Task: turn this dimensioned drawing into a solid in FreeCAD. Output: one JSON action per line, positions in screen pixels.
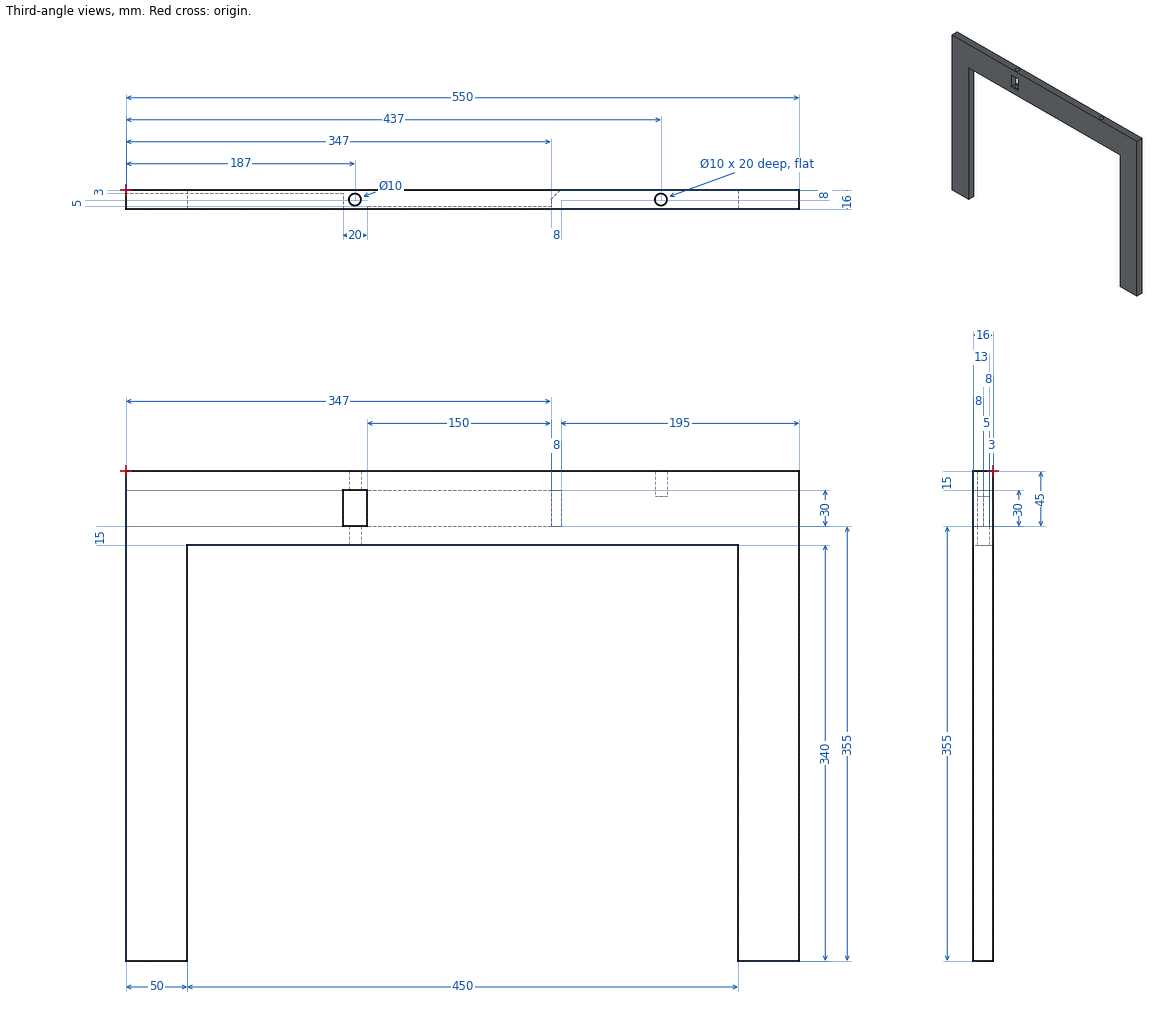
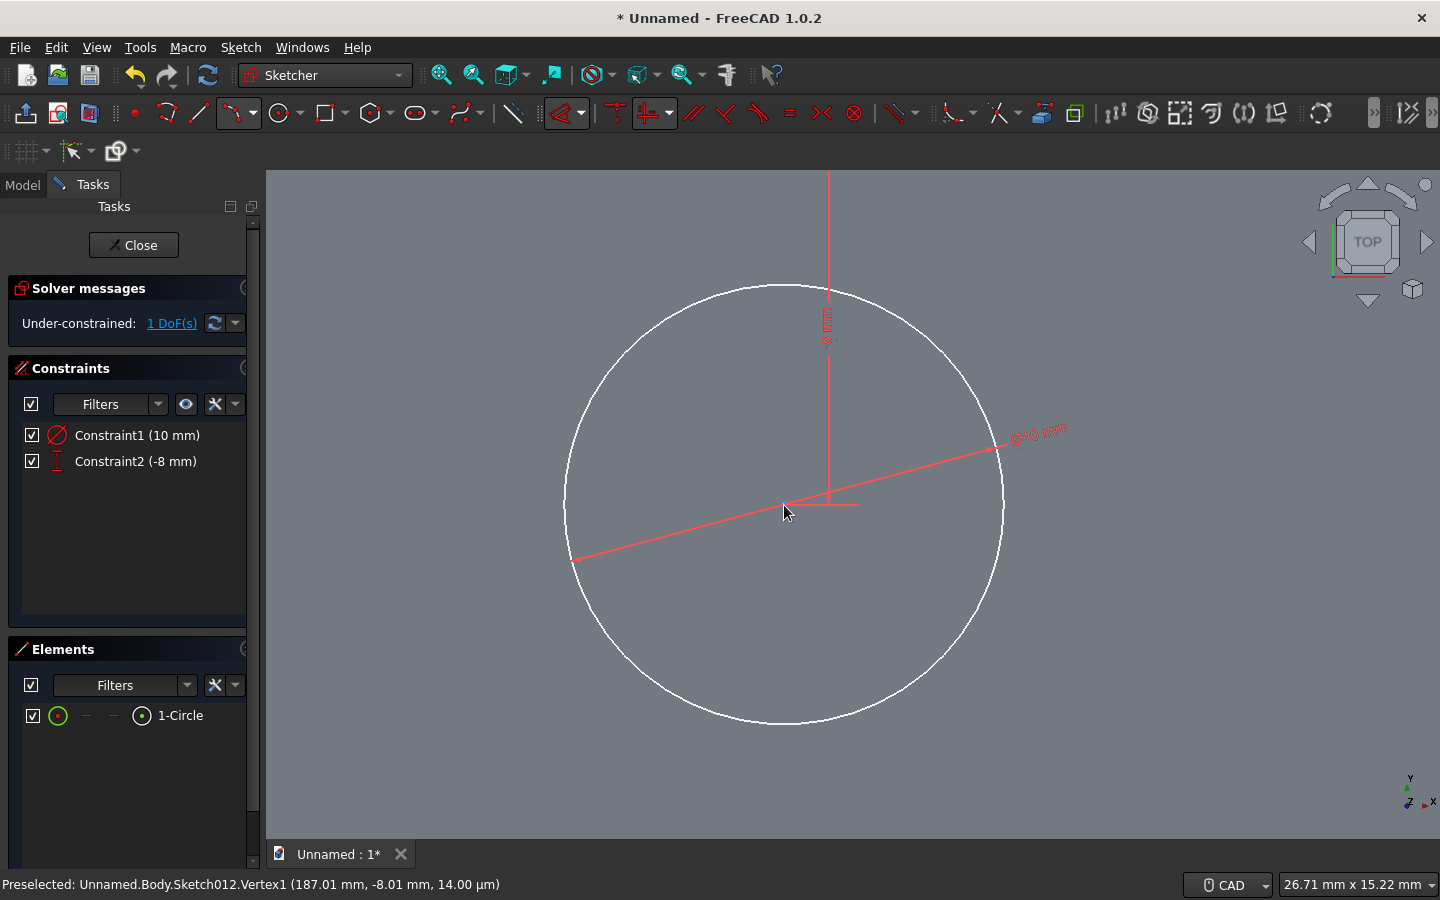
{"action": "left_click", "coordinate": [784, 504]}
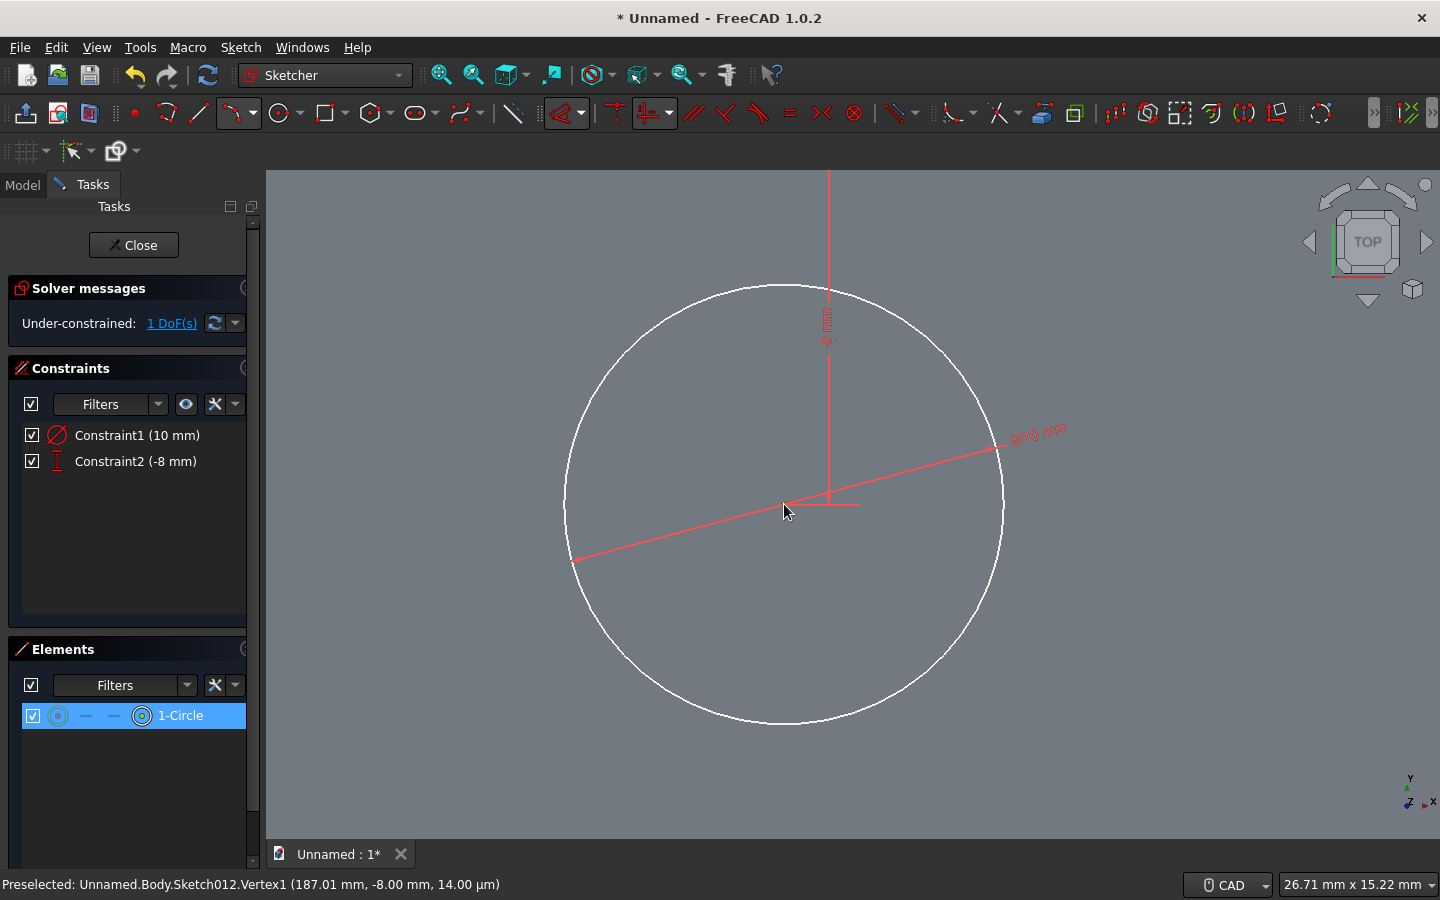
{"action": "key", "text": "l"}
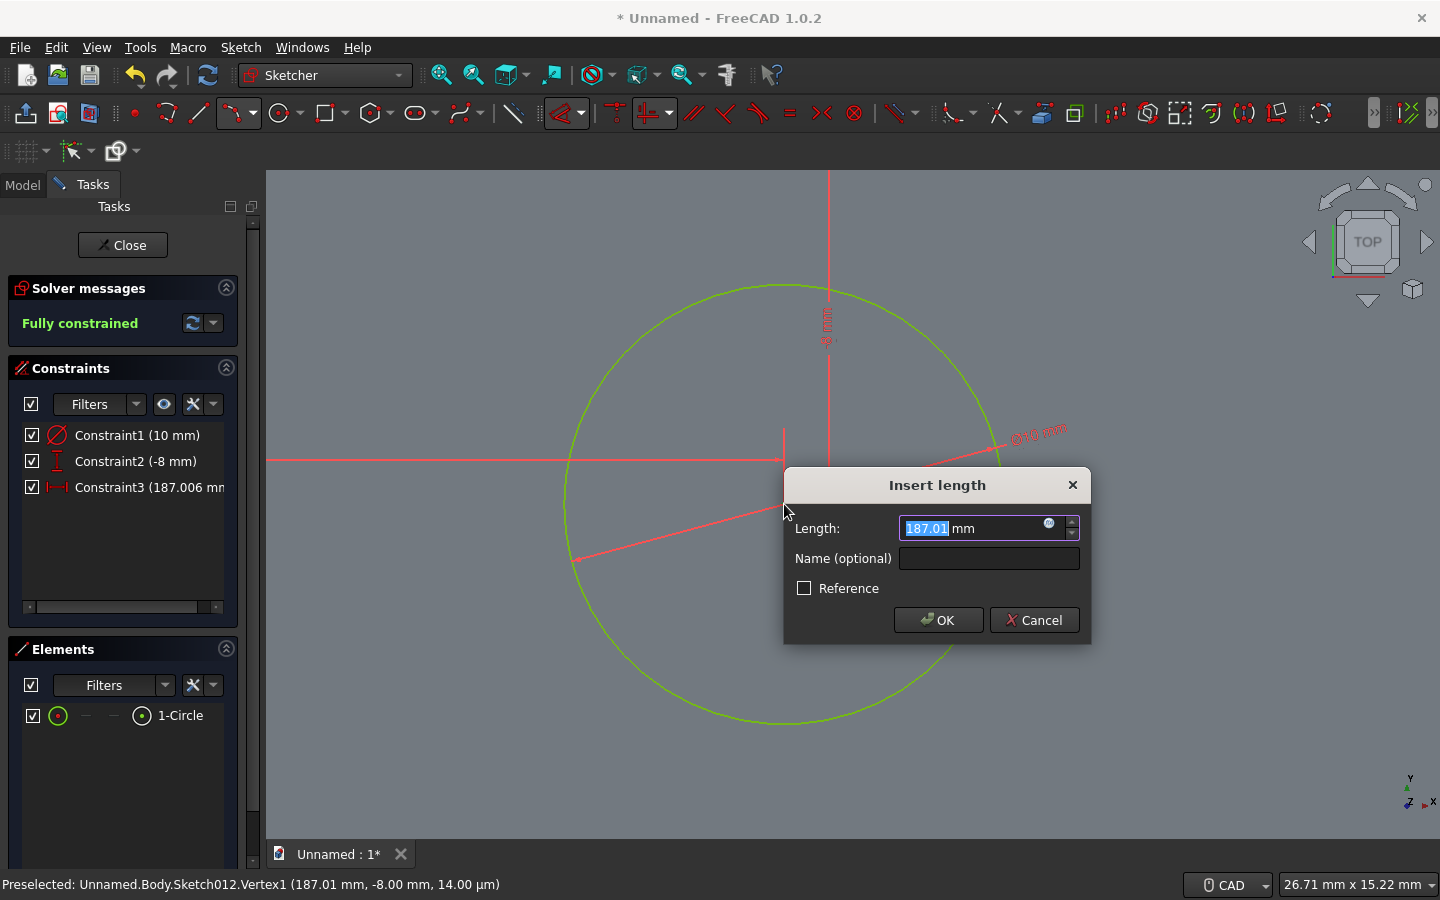
{"action": "type", "text": "187"}
{"action": "key", "text": "Return"}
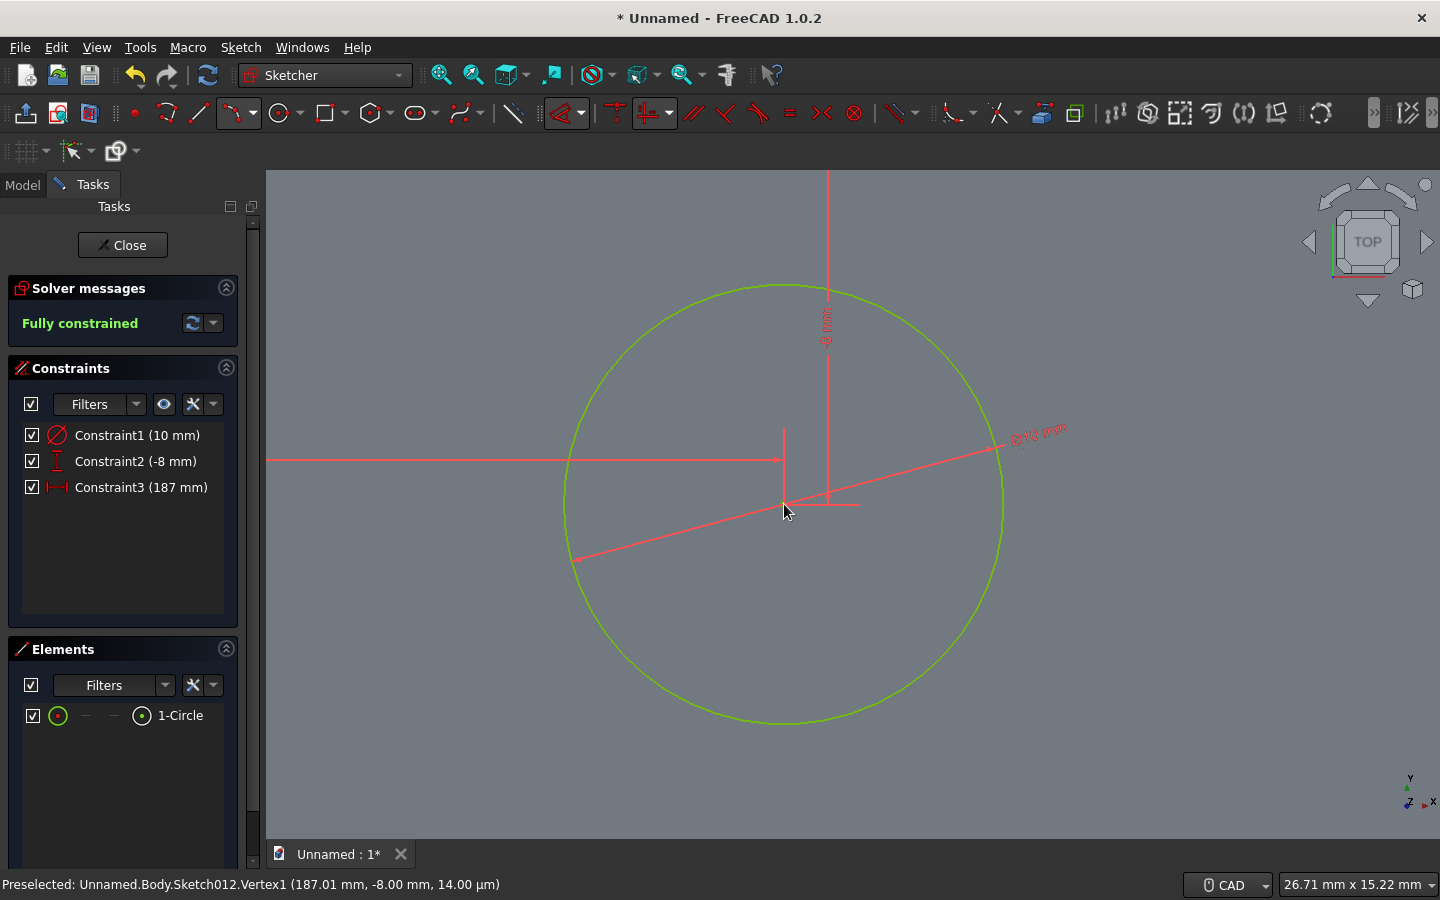
{"action": "left_click", "coordinate": [123, 245]}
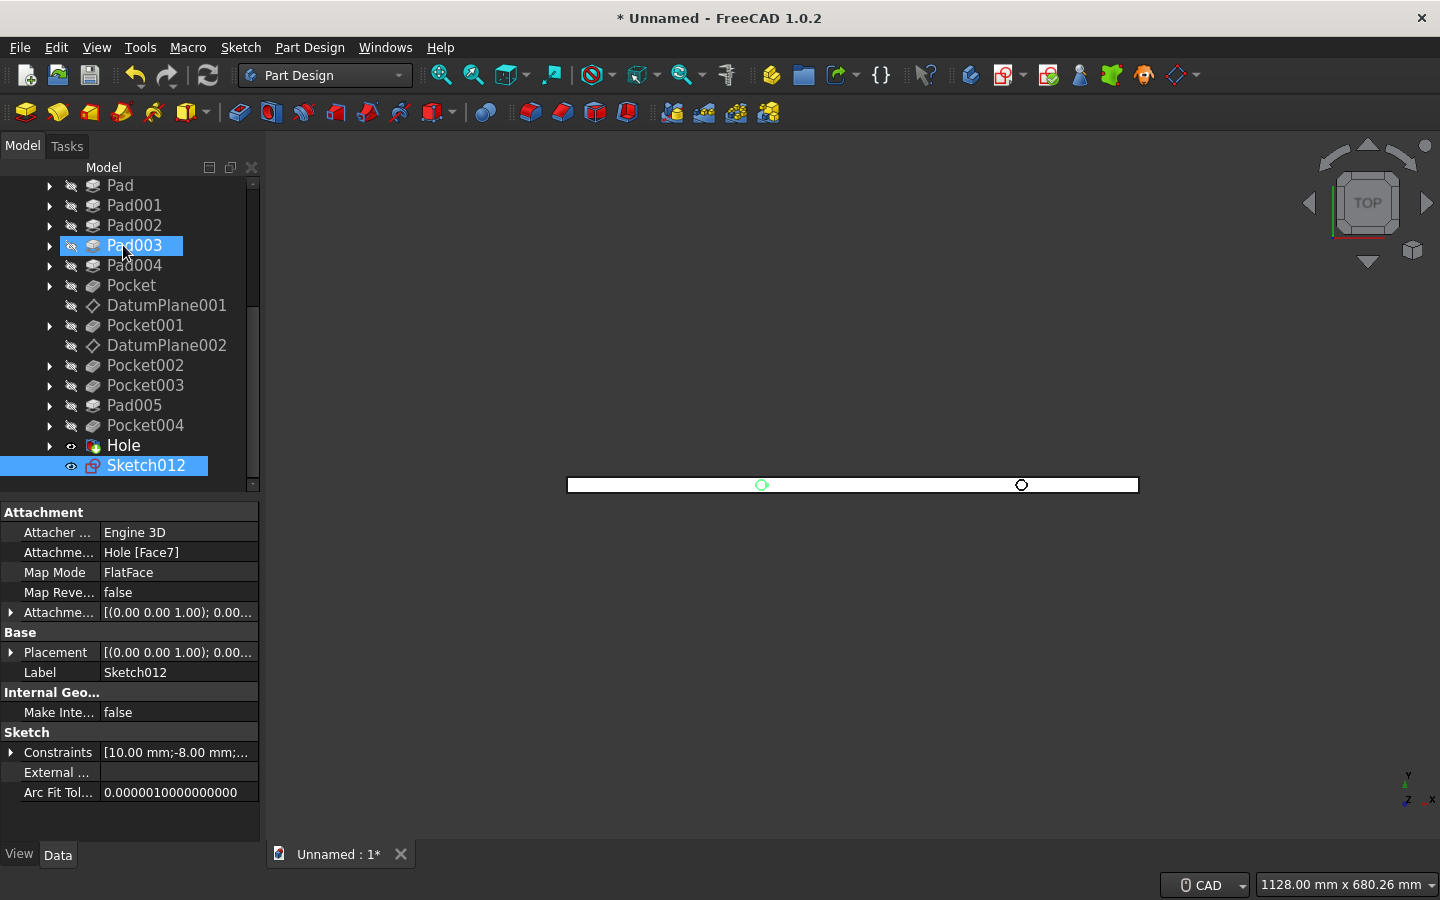
{"action": "left_click", "coordinate": [240, 112]}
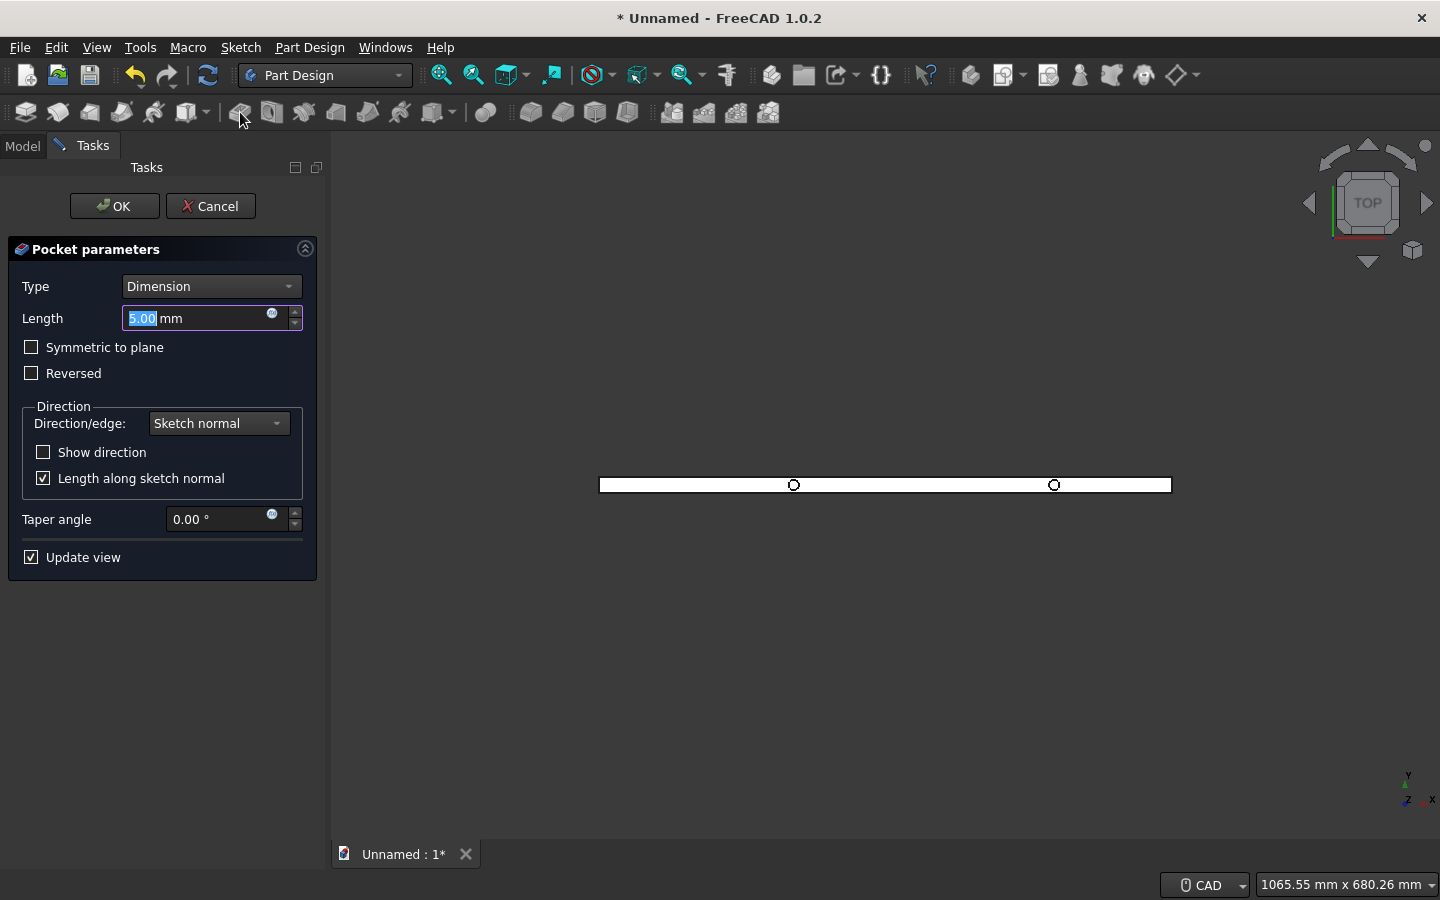
{"action": "type", "text": "15"}
{"action": "key", "text": "Tab"}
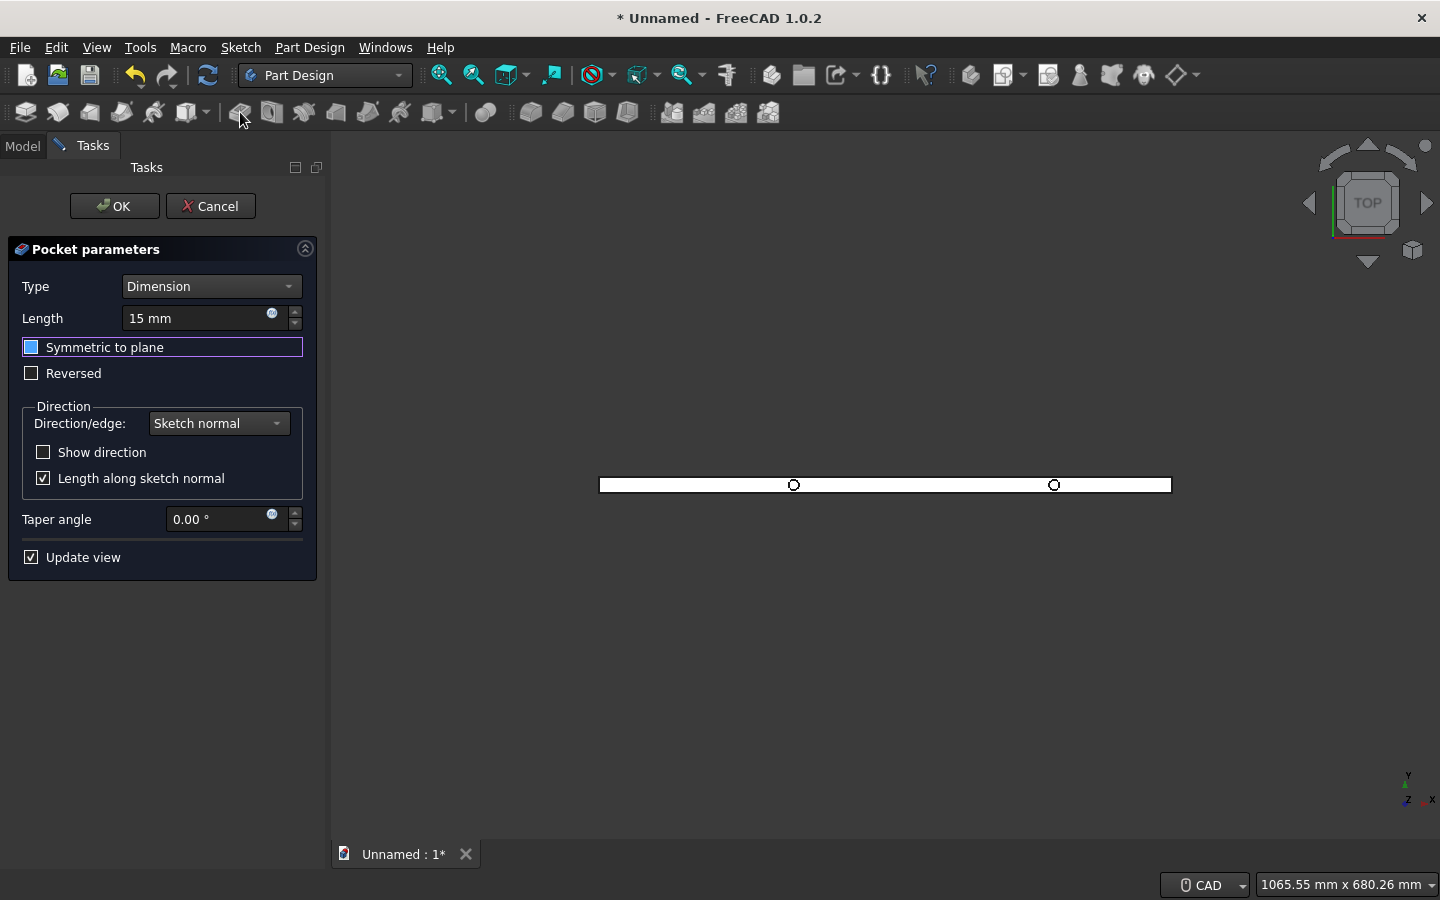
{"action": "left_click", "coordinate": [115, 206]}